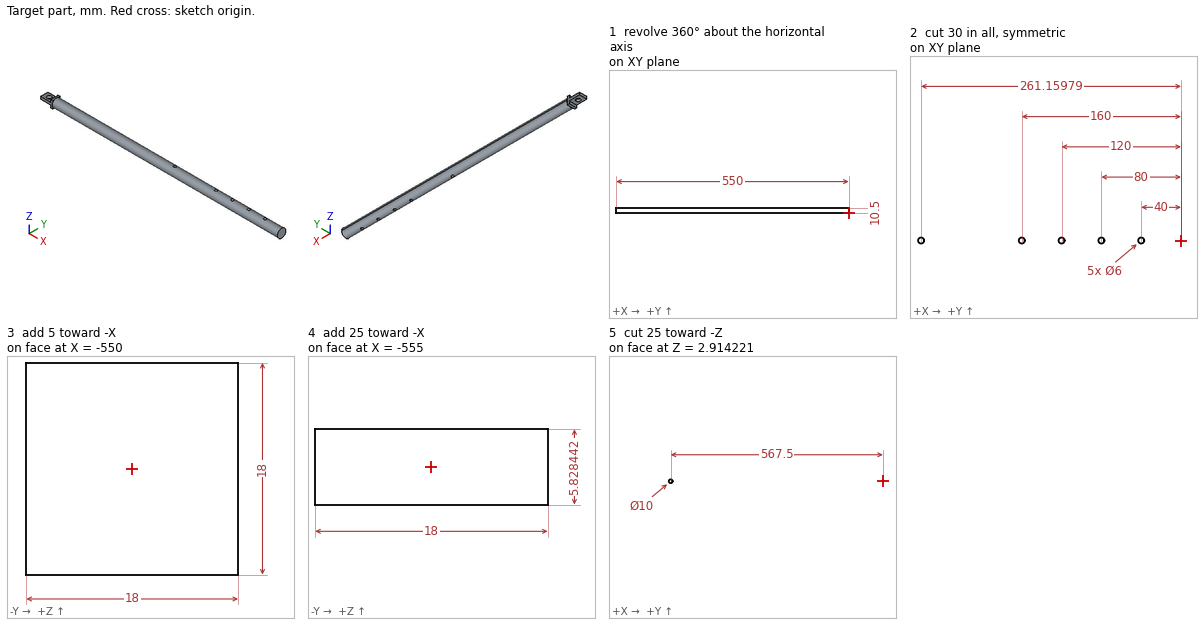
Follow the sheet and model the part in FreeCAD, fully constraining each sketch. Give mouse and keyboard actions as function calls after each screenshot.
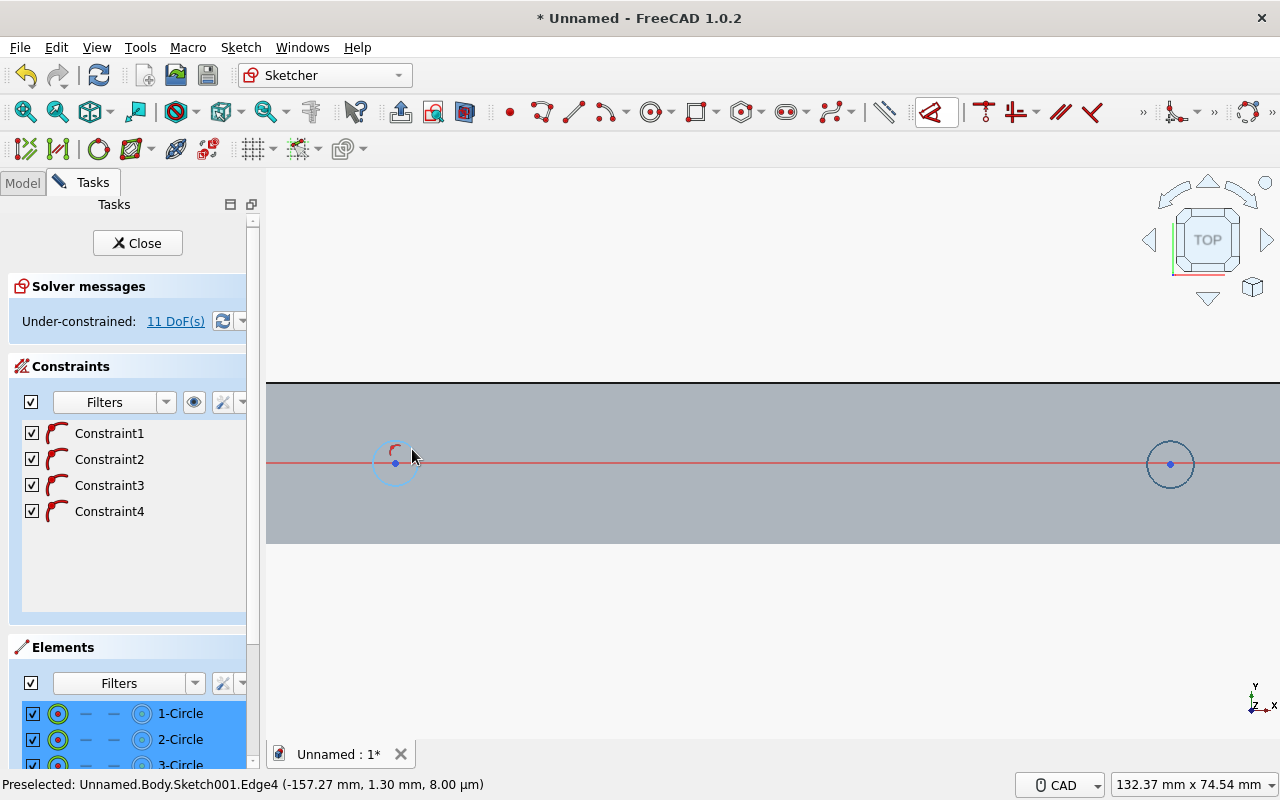
click(411, 447)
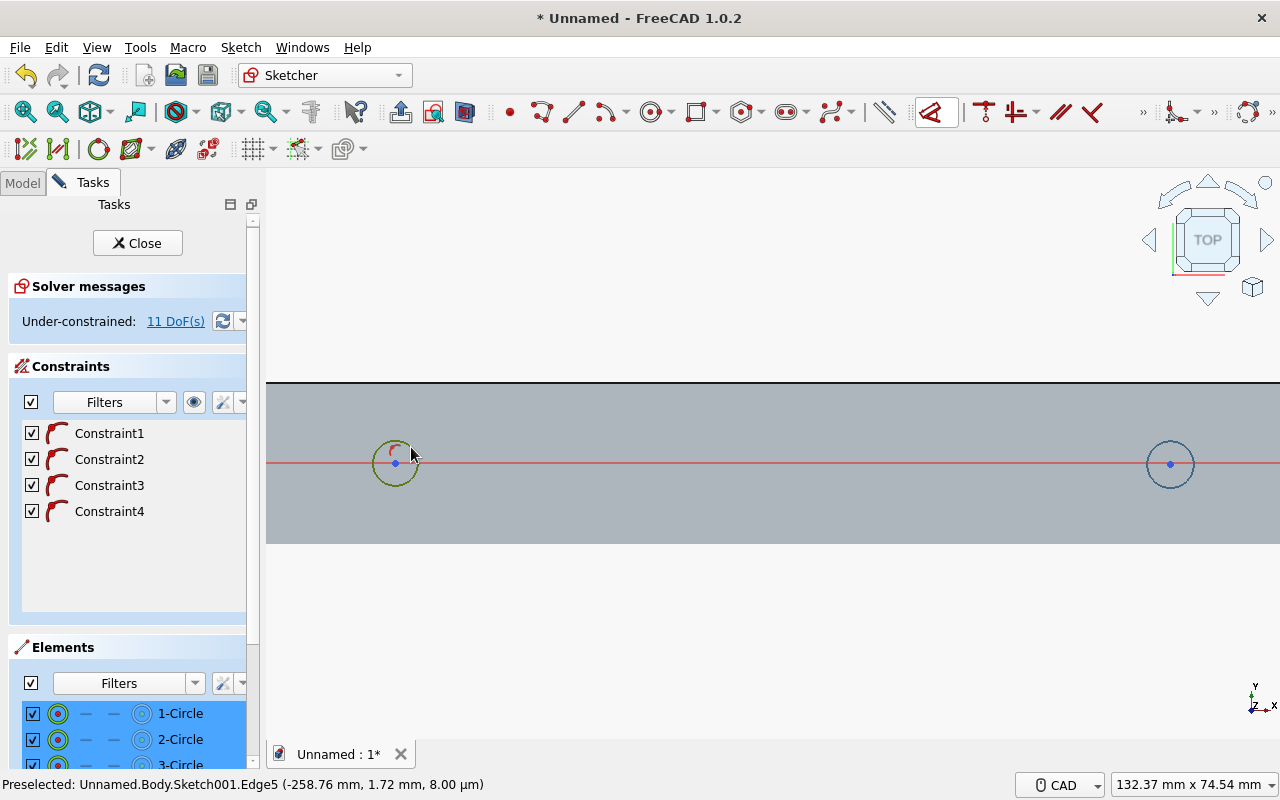
key(e)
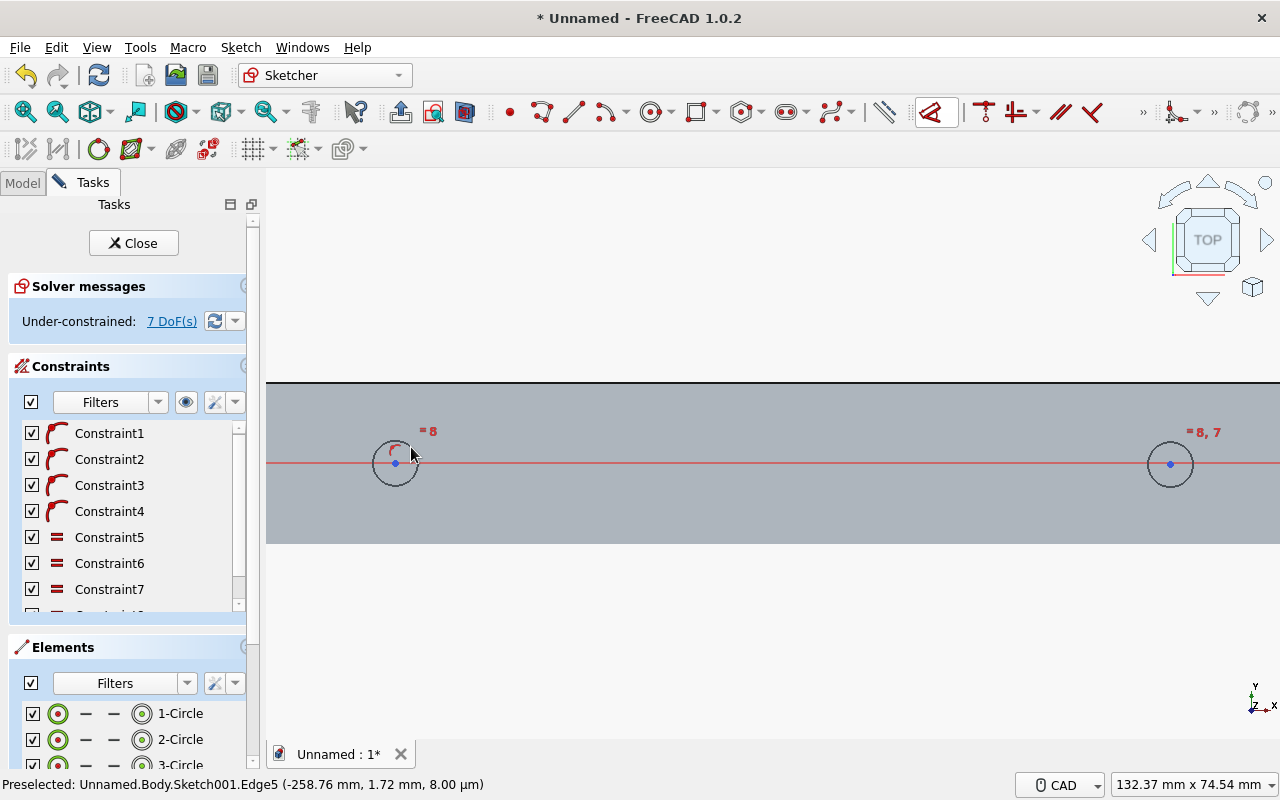
scroll(412, 449, down, 6)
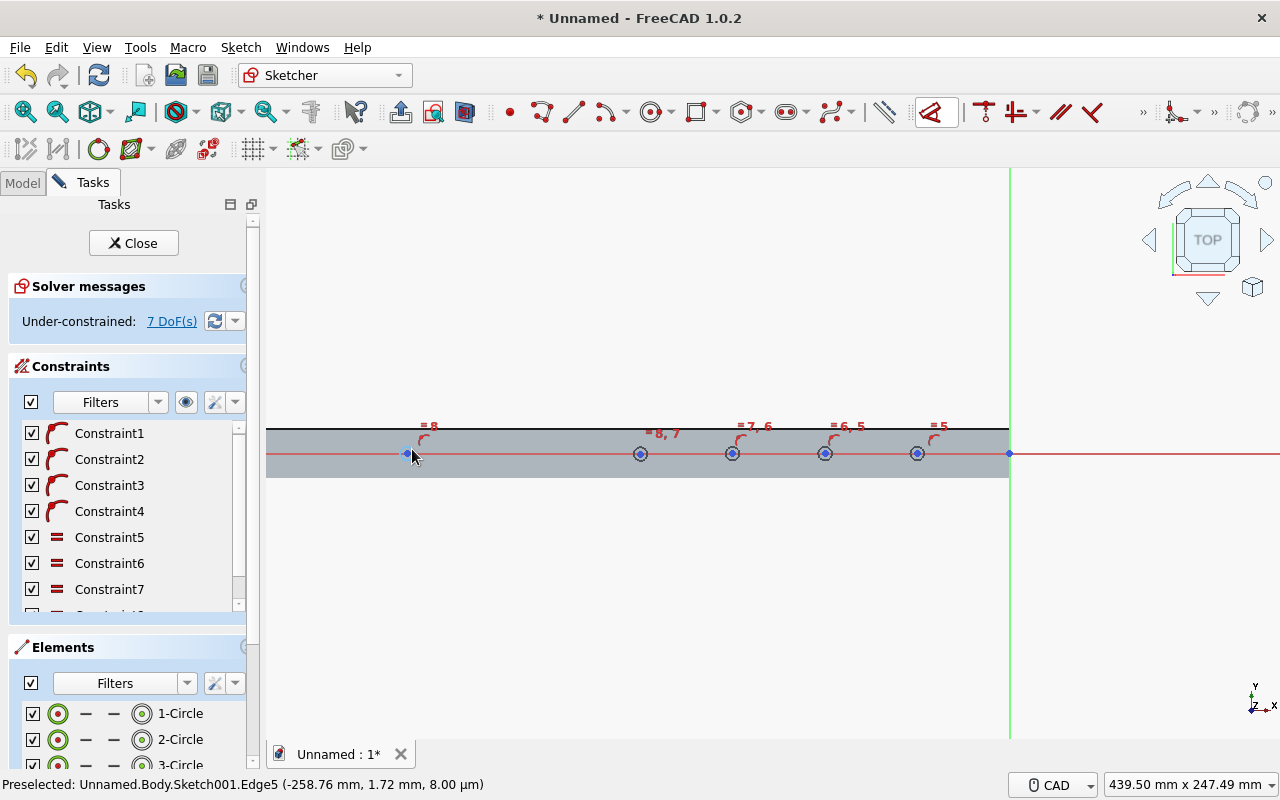
click(641, 454)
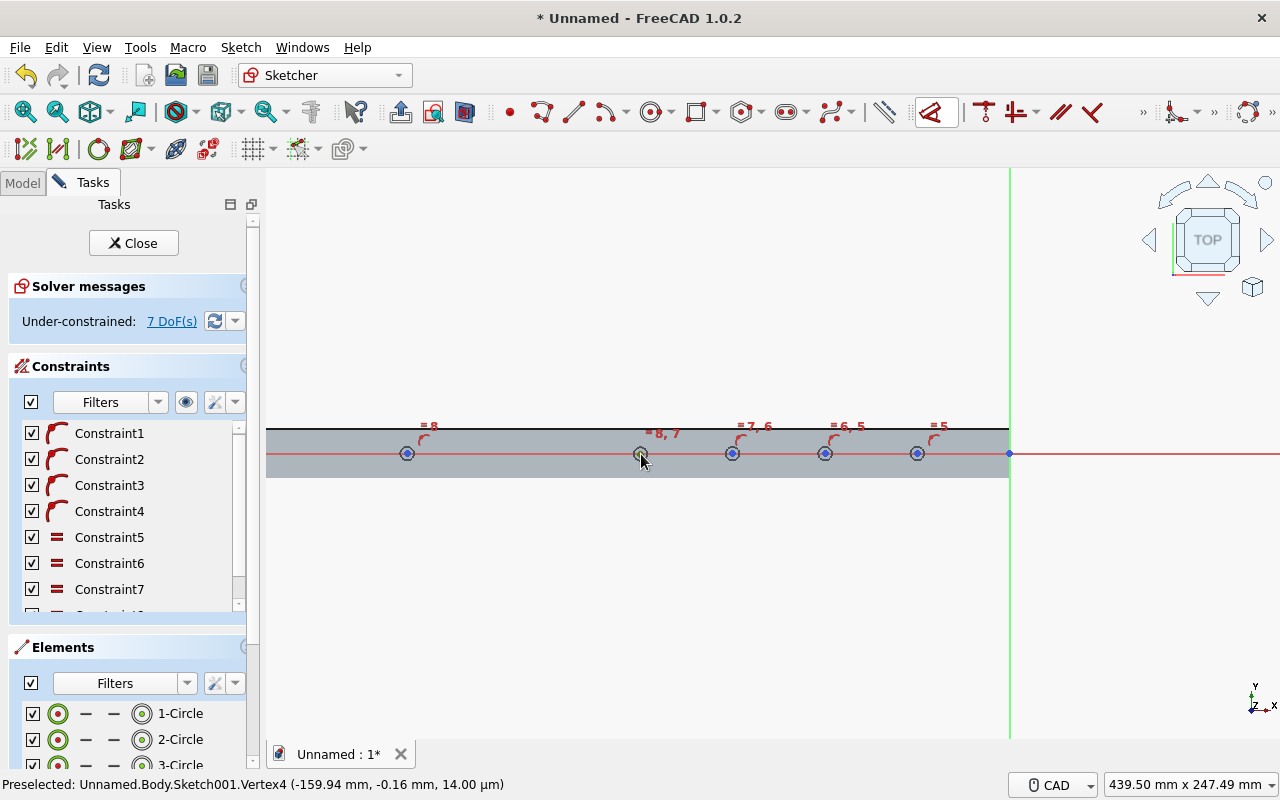
click(353, 454)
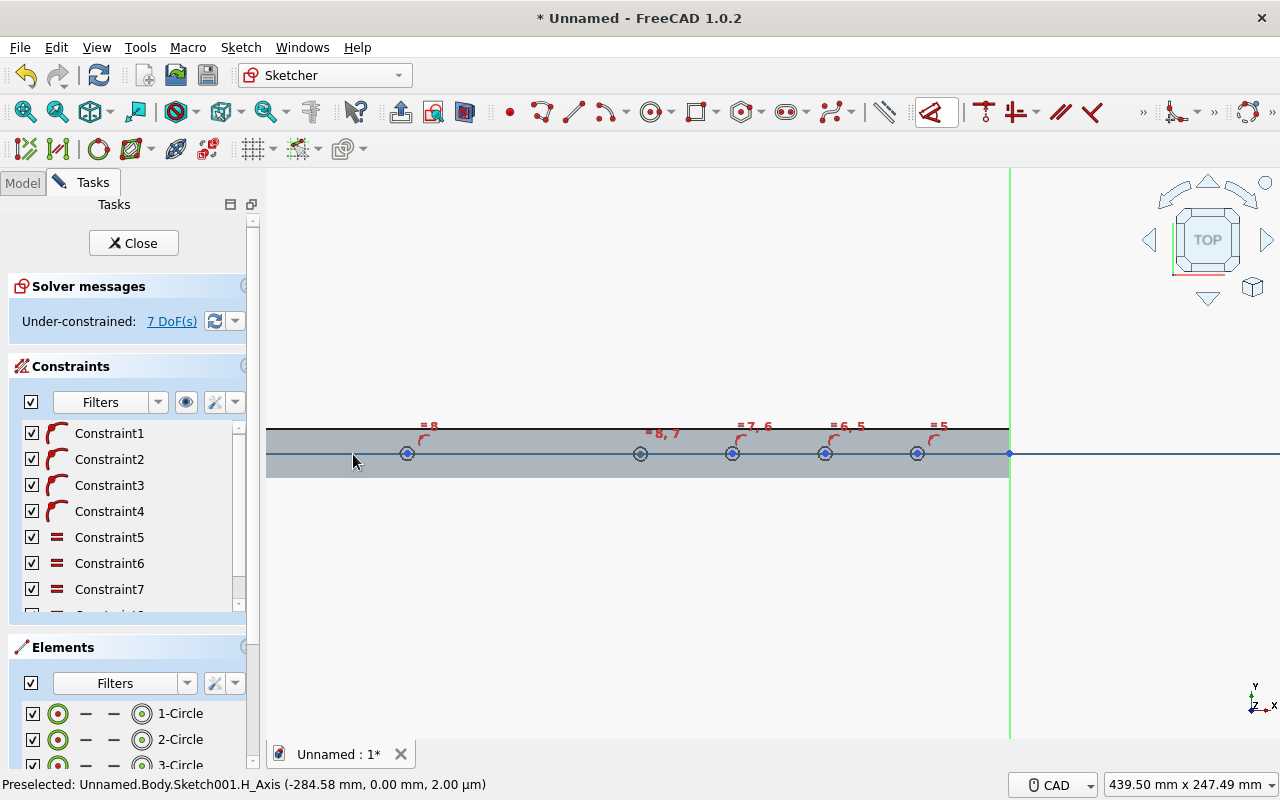
click(984, 112)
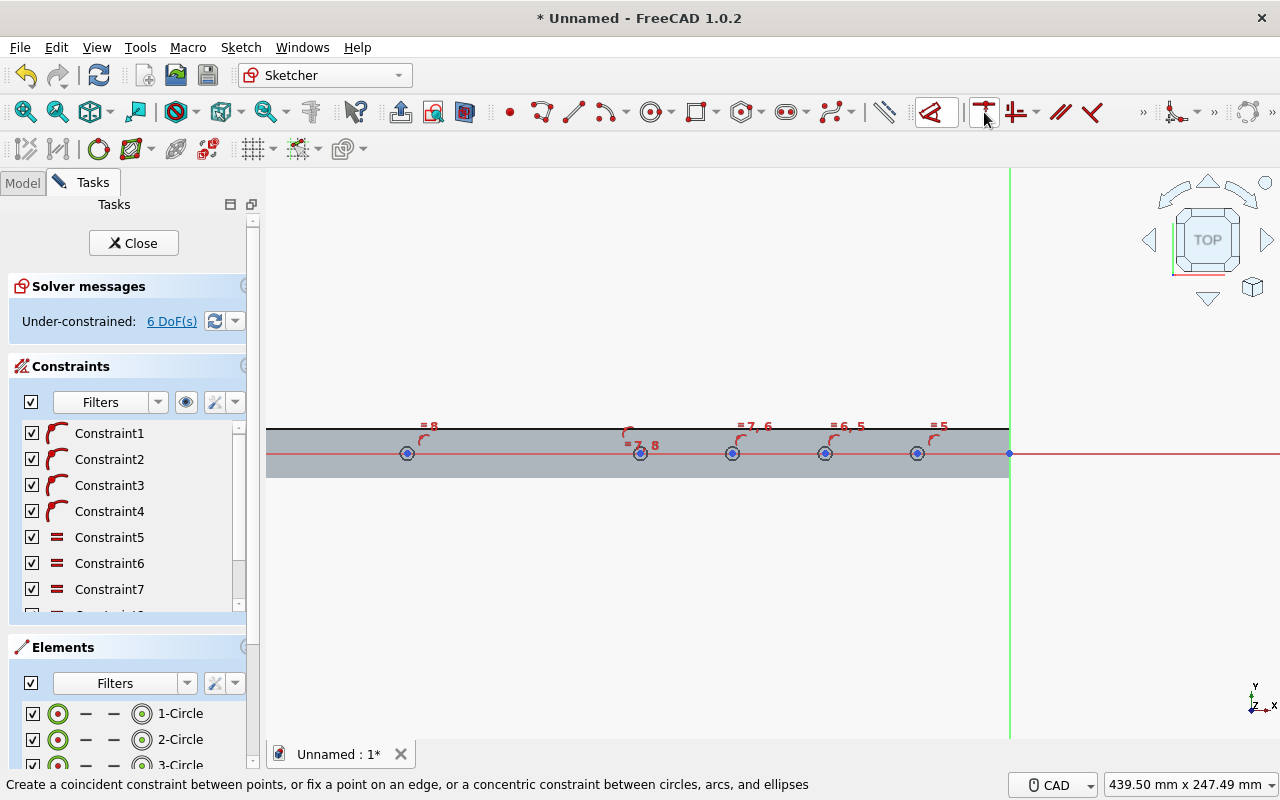
key(d)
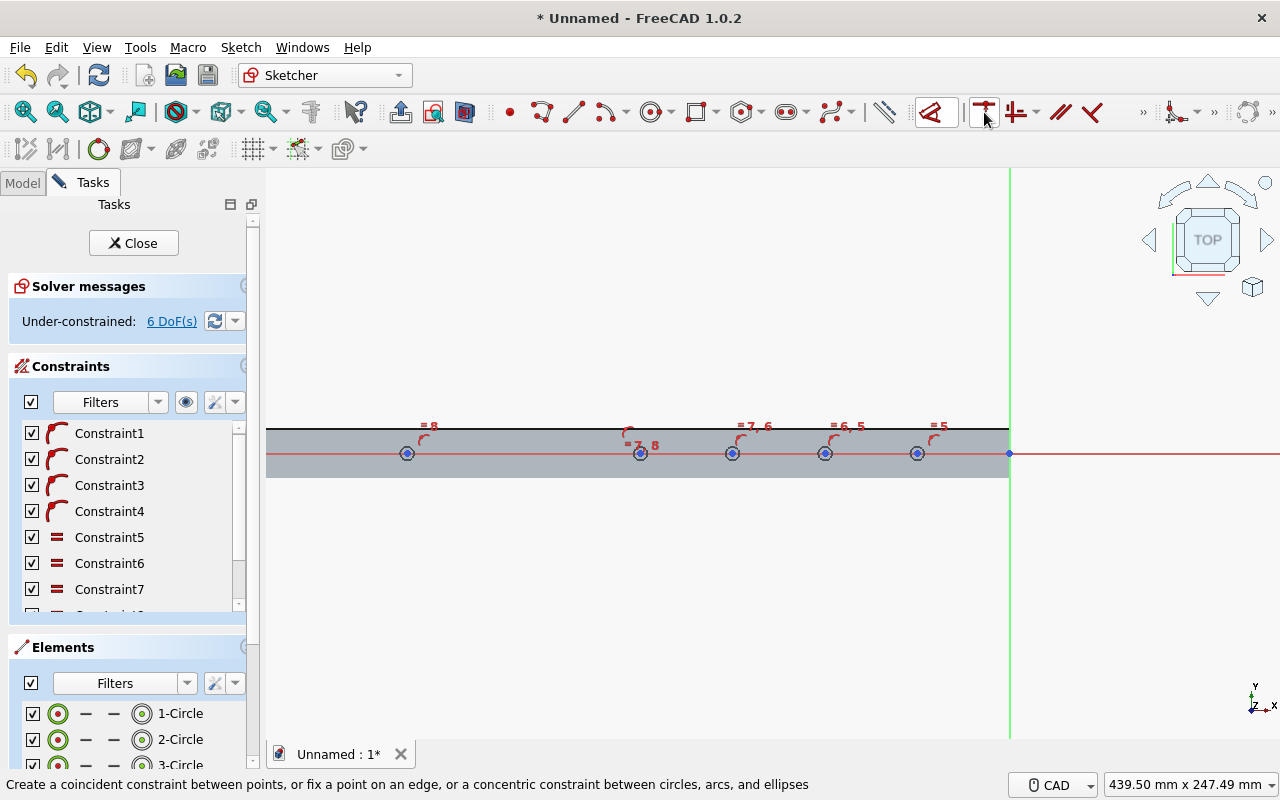
scroll(910, 453, up, 6)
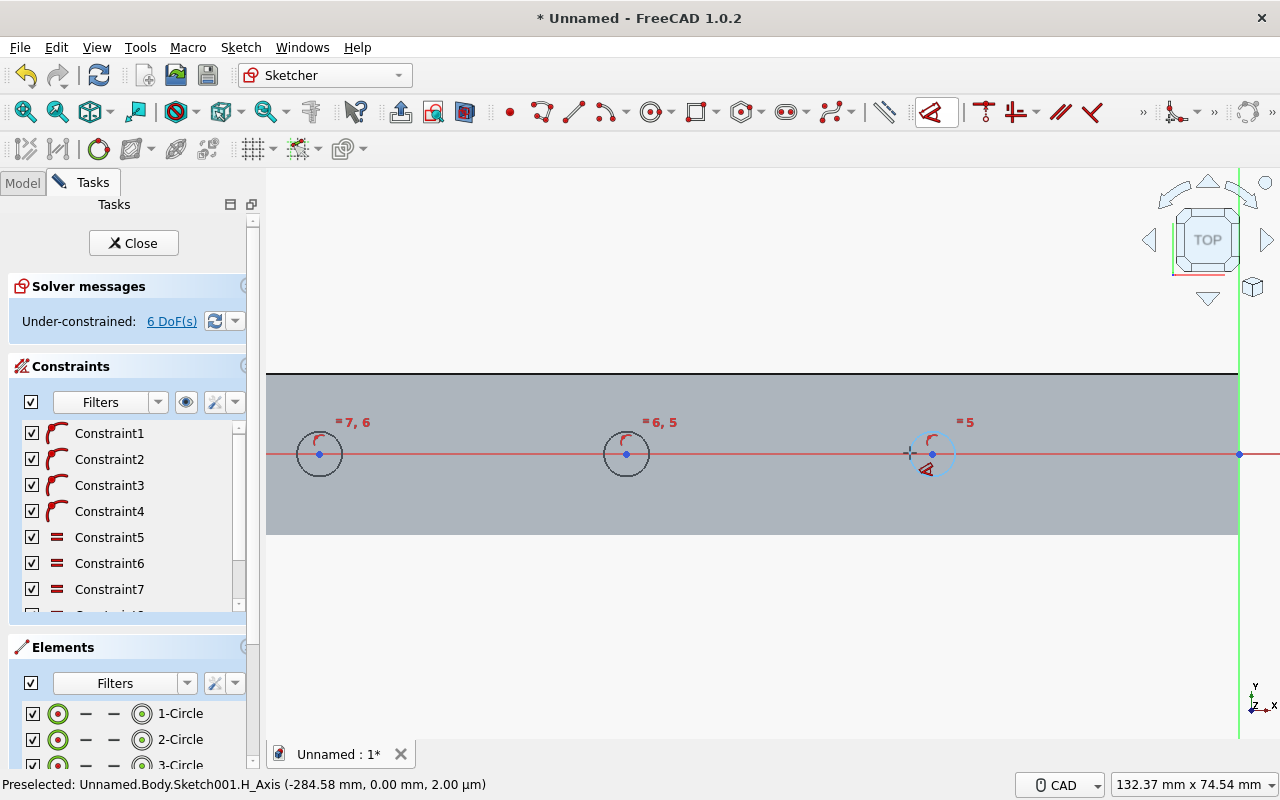
click(910, 453)
click(886, 426)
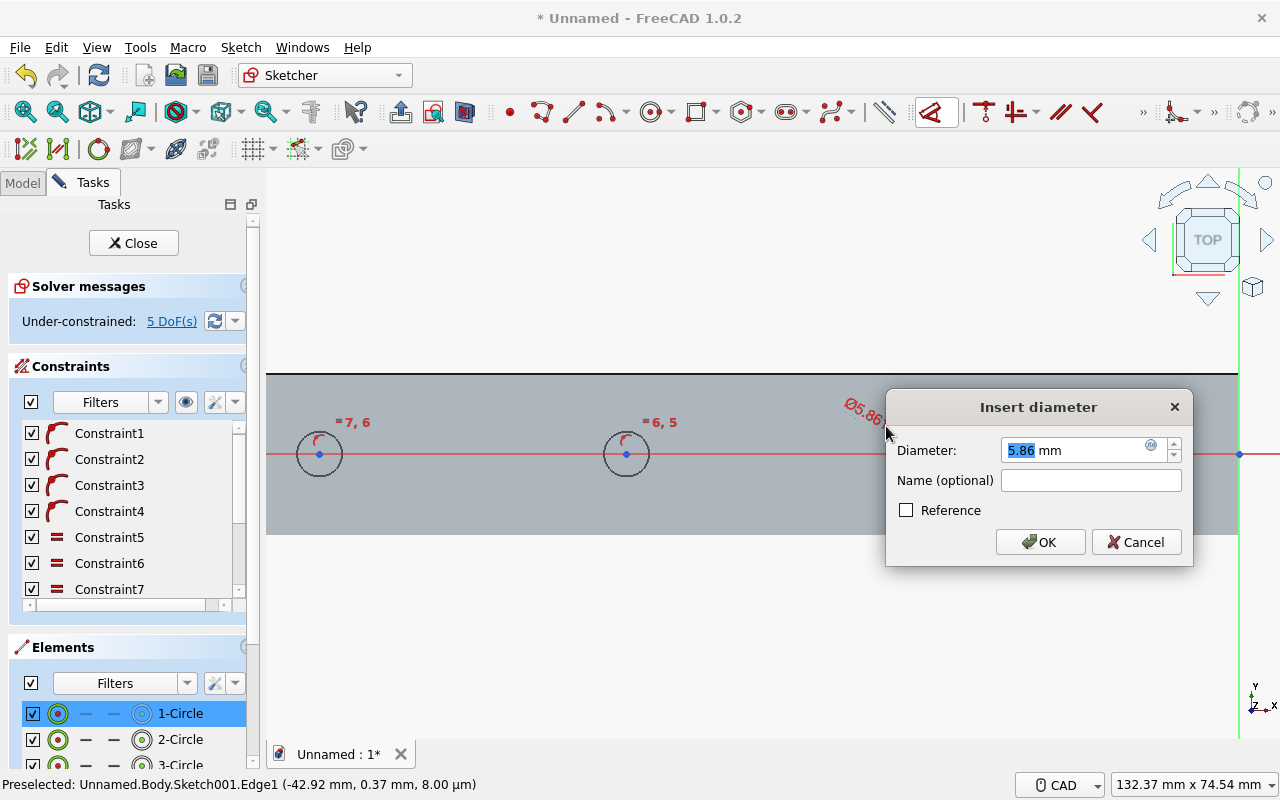
text(6)
key(Return)